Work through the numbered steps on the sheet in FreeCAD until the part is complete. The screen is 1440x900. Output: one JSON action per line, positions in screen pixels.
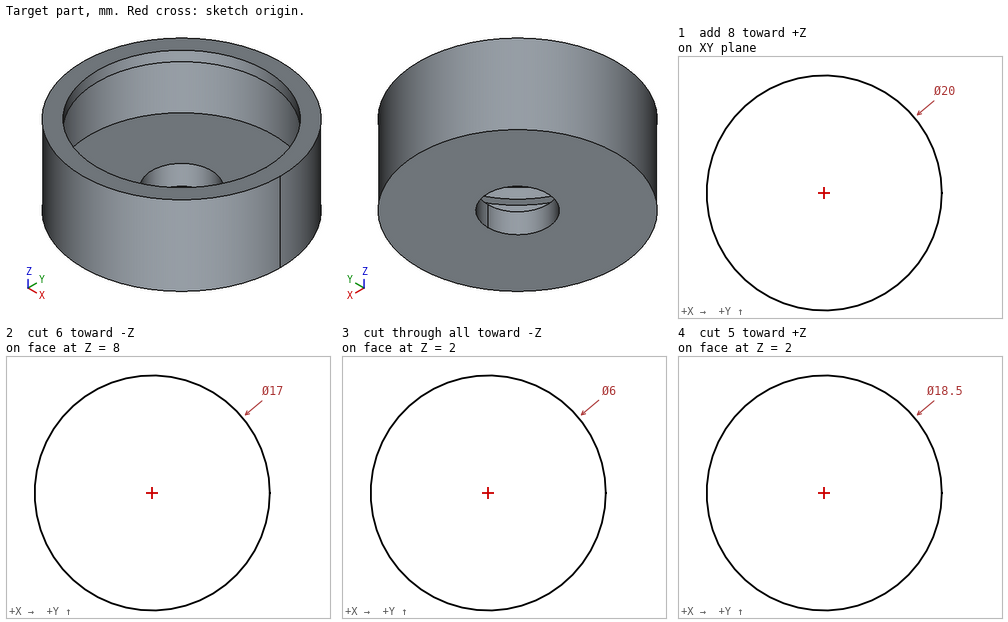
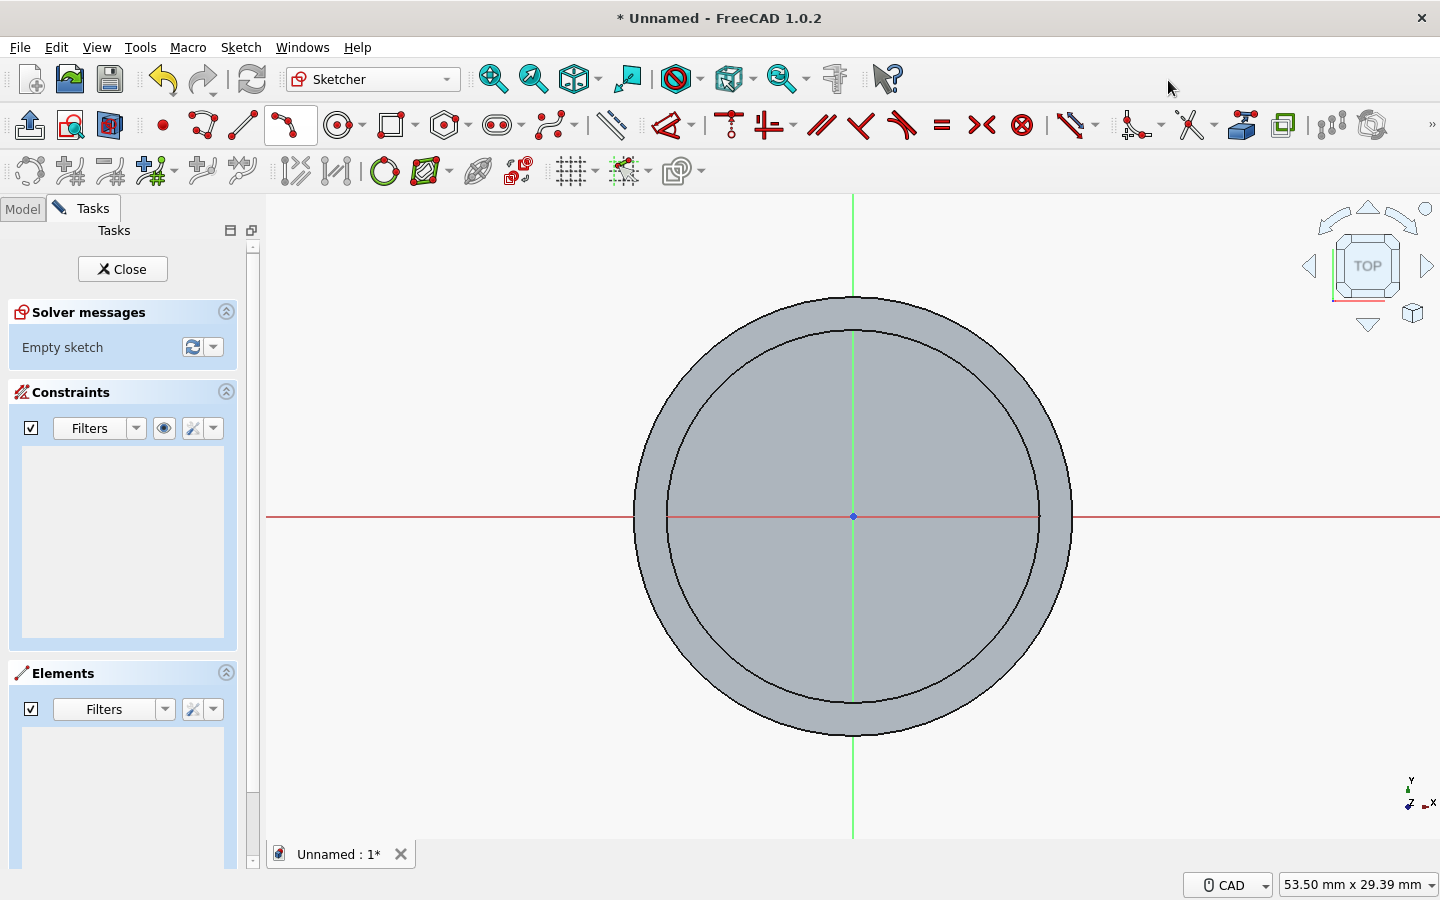
{"action": "scroll", "coordinate": [883, 516], "scroll_direction": "up", "scroll_amount": 6}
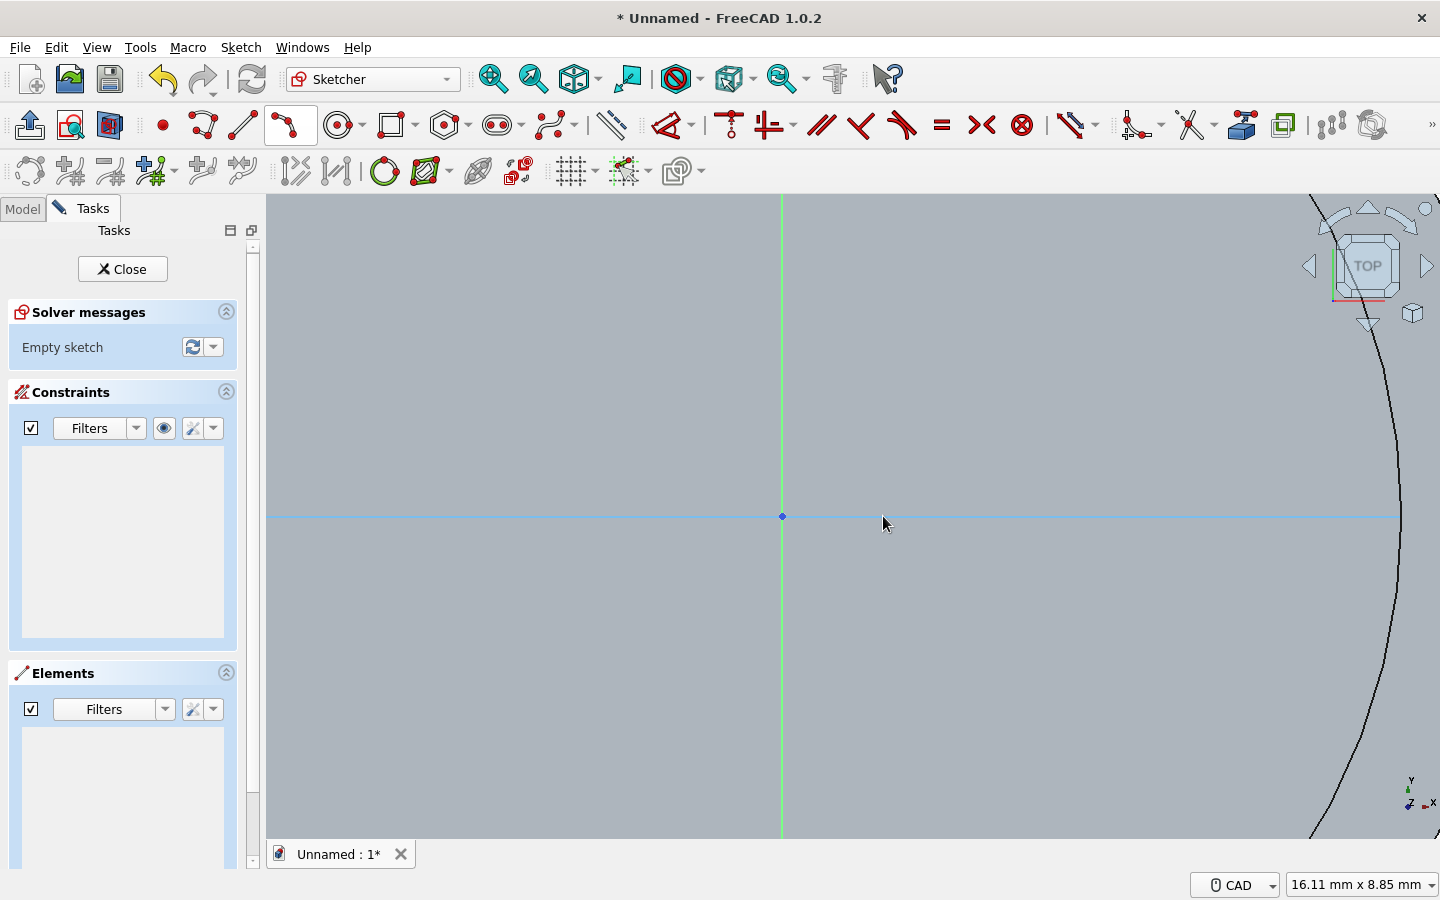
{"action": "left_click", "coordinate": [338, 126]}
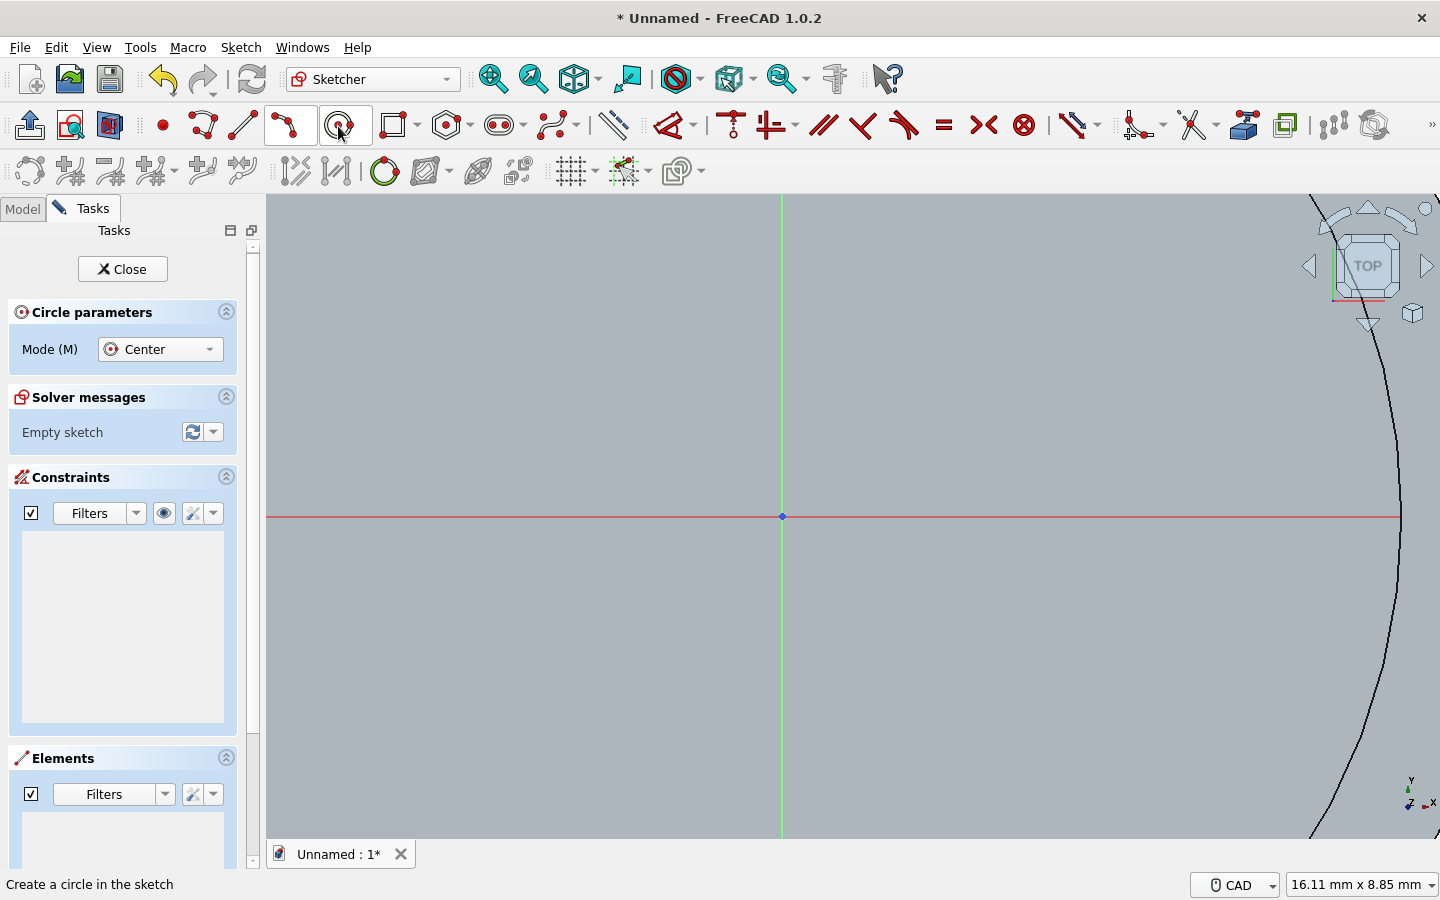
{"action": "left_click", "coordinate": [782, 516]}
{"action": "mouse_move", "coordinate": [937, 362]}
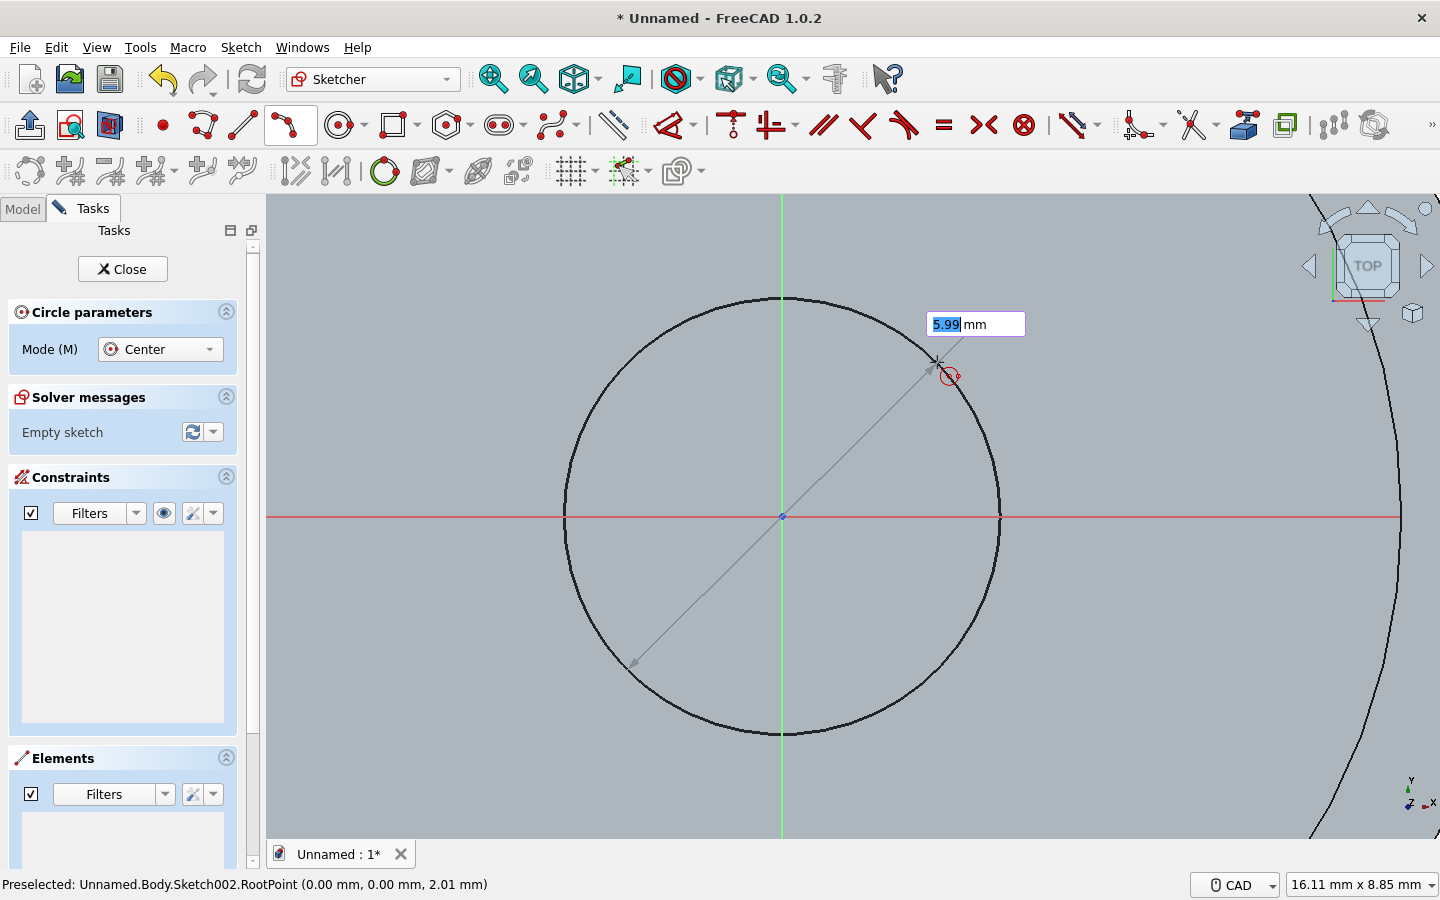
{"action": "type", "text": "6"}
{"action": "key", "text": "Return"}
{"action": "key", "text": "Escape"}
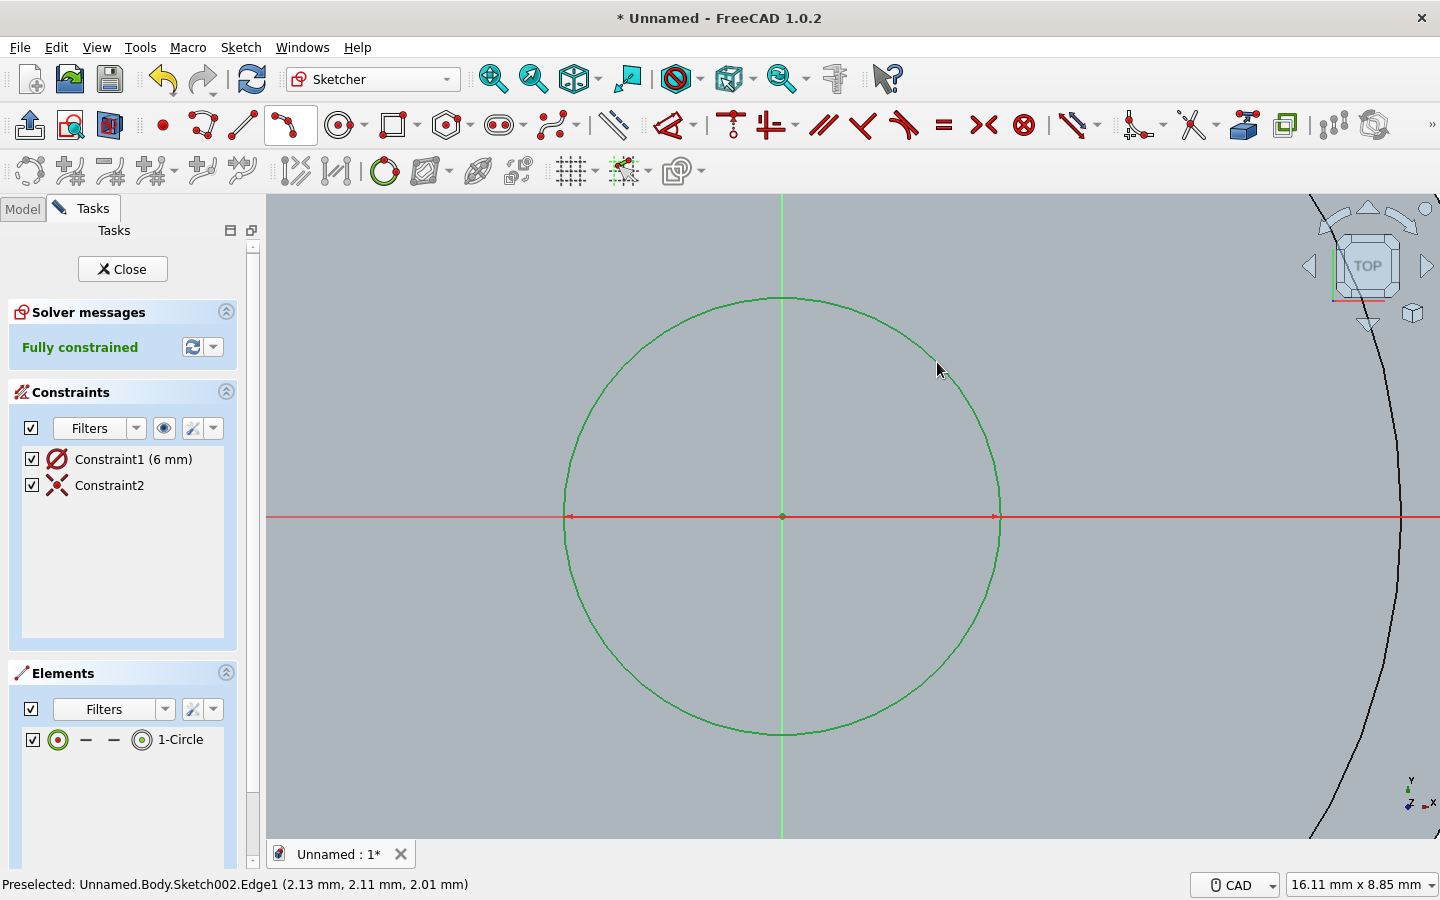
{"action": "left_click", "coordinate": [123, 269]}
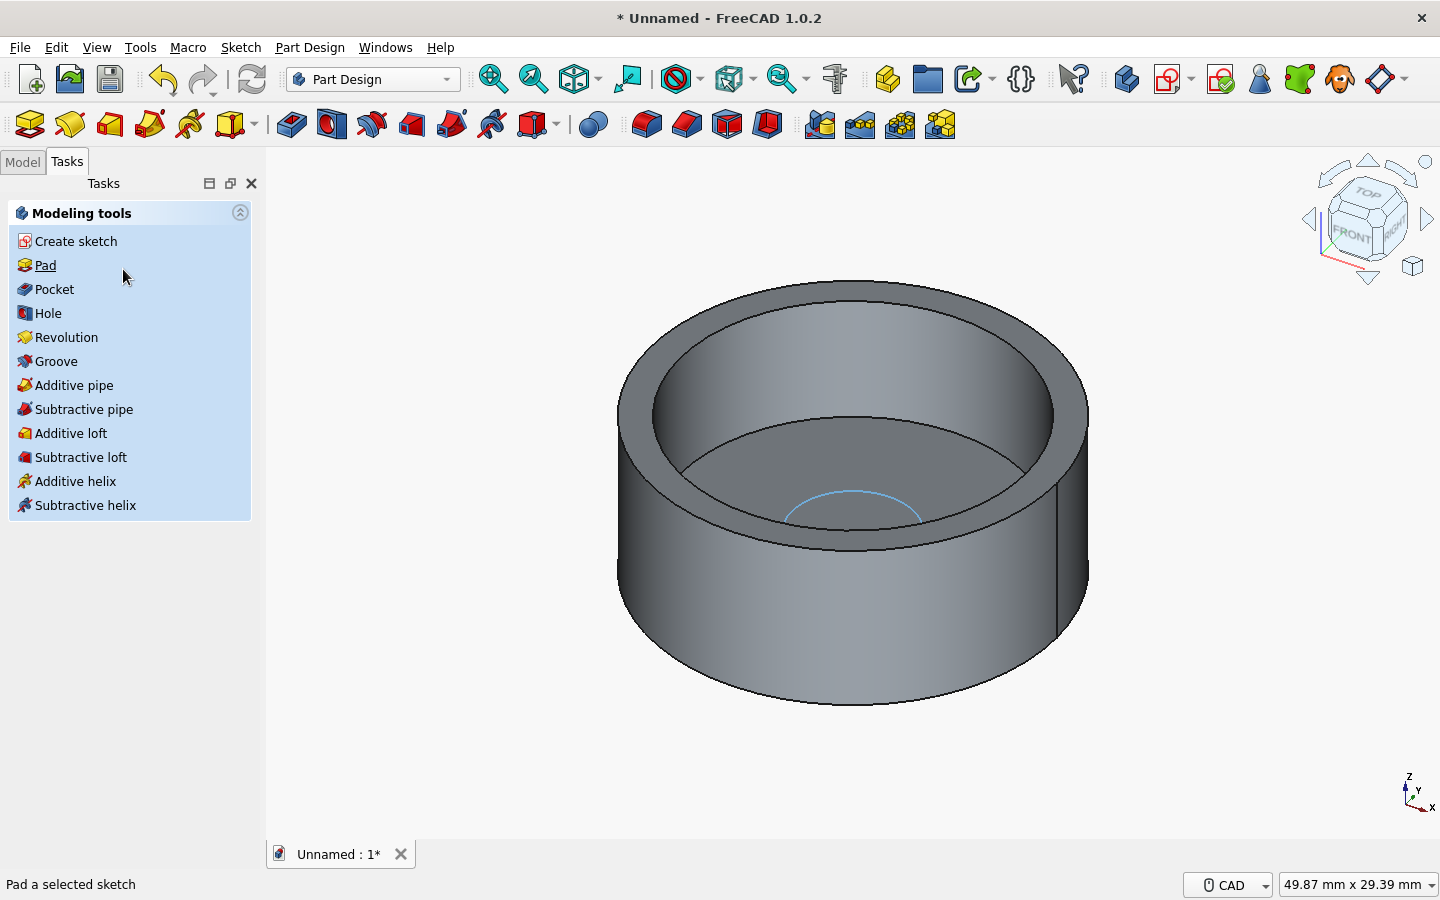
{"action": "left_click", "coordinate": [292, 124]}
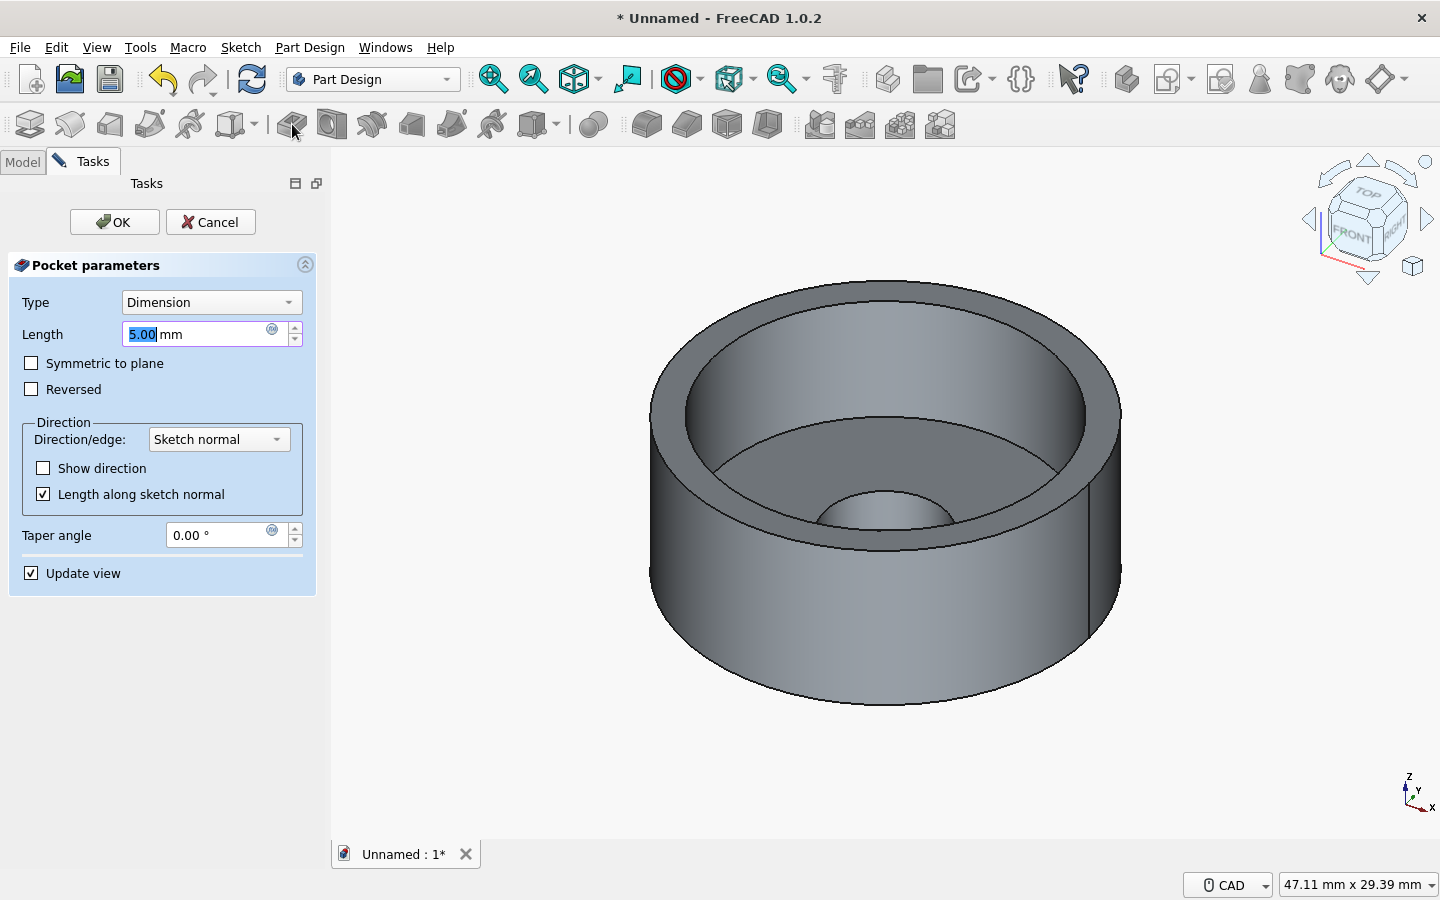
{"action": "left_click", "coordinate": [212, 302]}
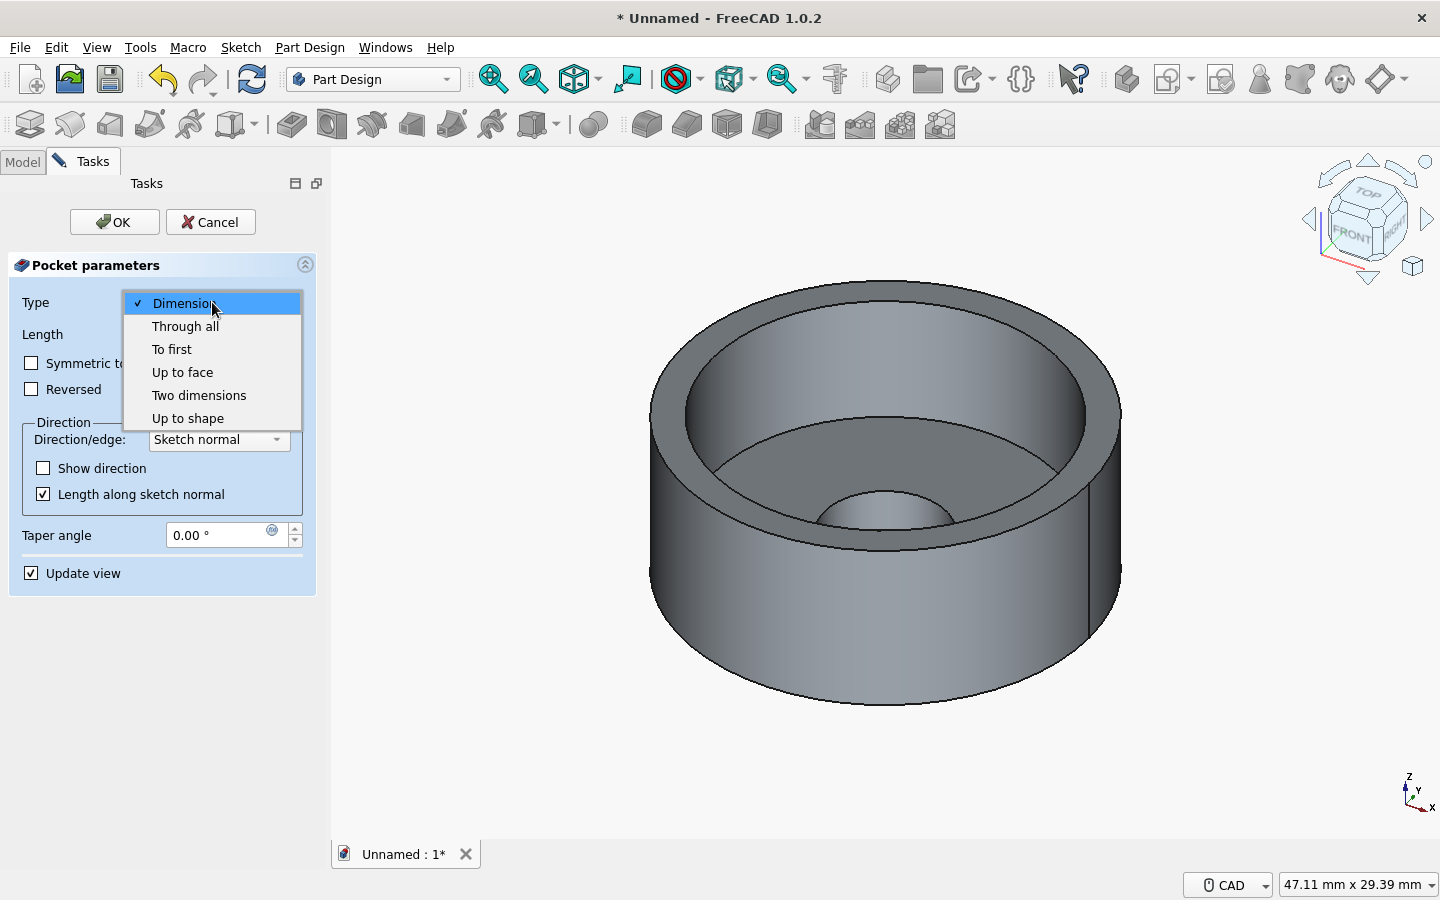
{"action": "left_click", "coordinate": [212, 326]}